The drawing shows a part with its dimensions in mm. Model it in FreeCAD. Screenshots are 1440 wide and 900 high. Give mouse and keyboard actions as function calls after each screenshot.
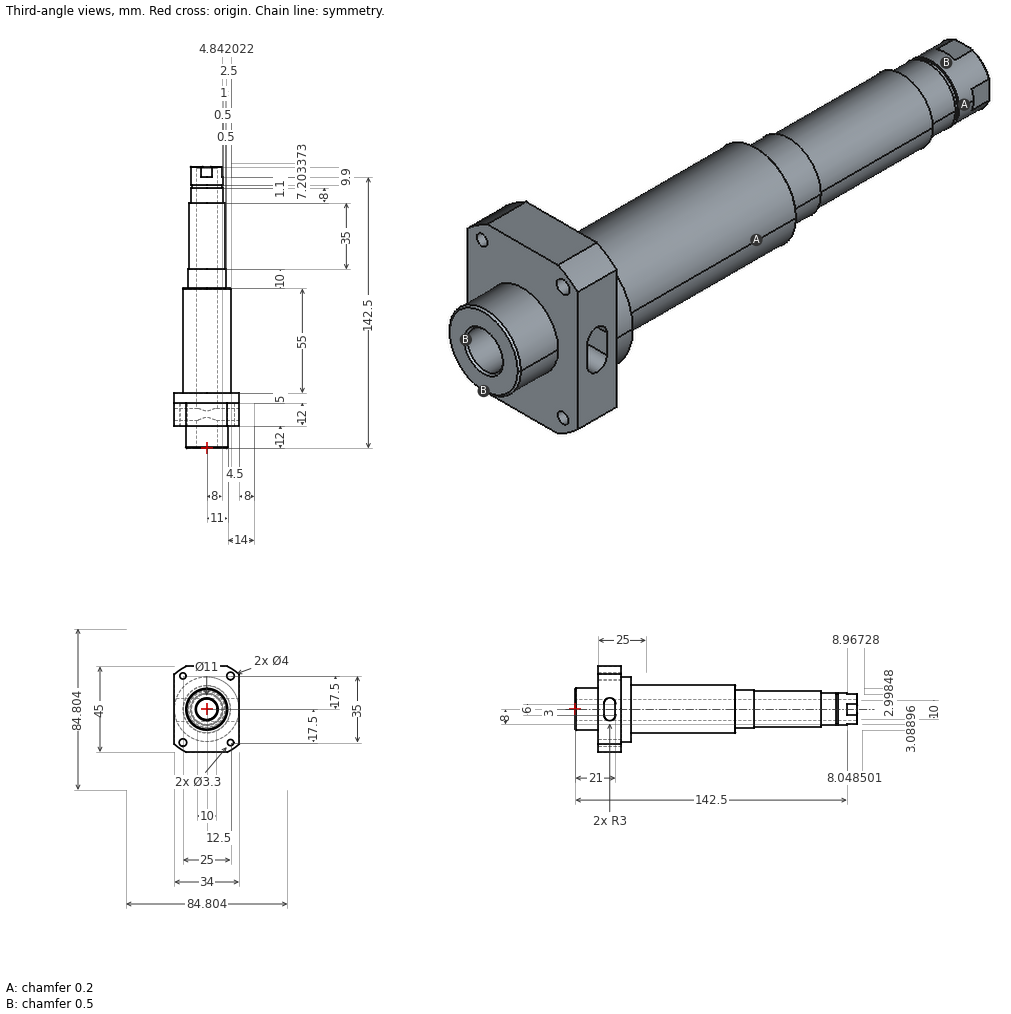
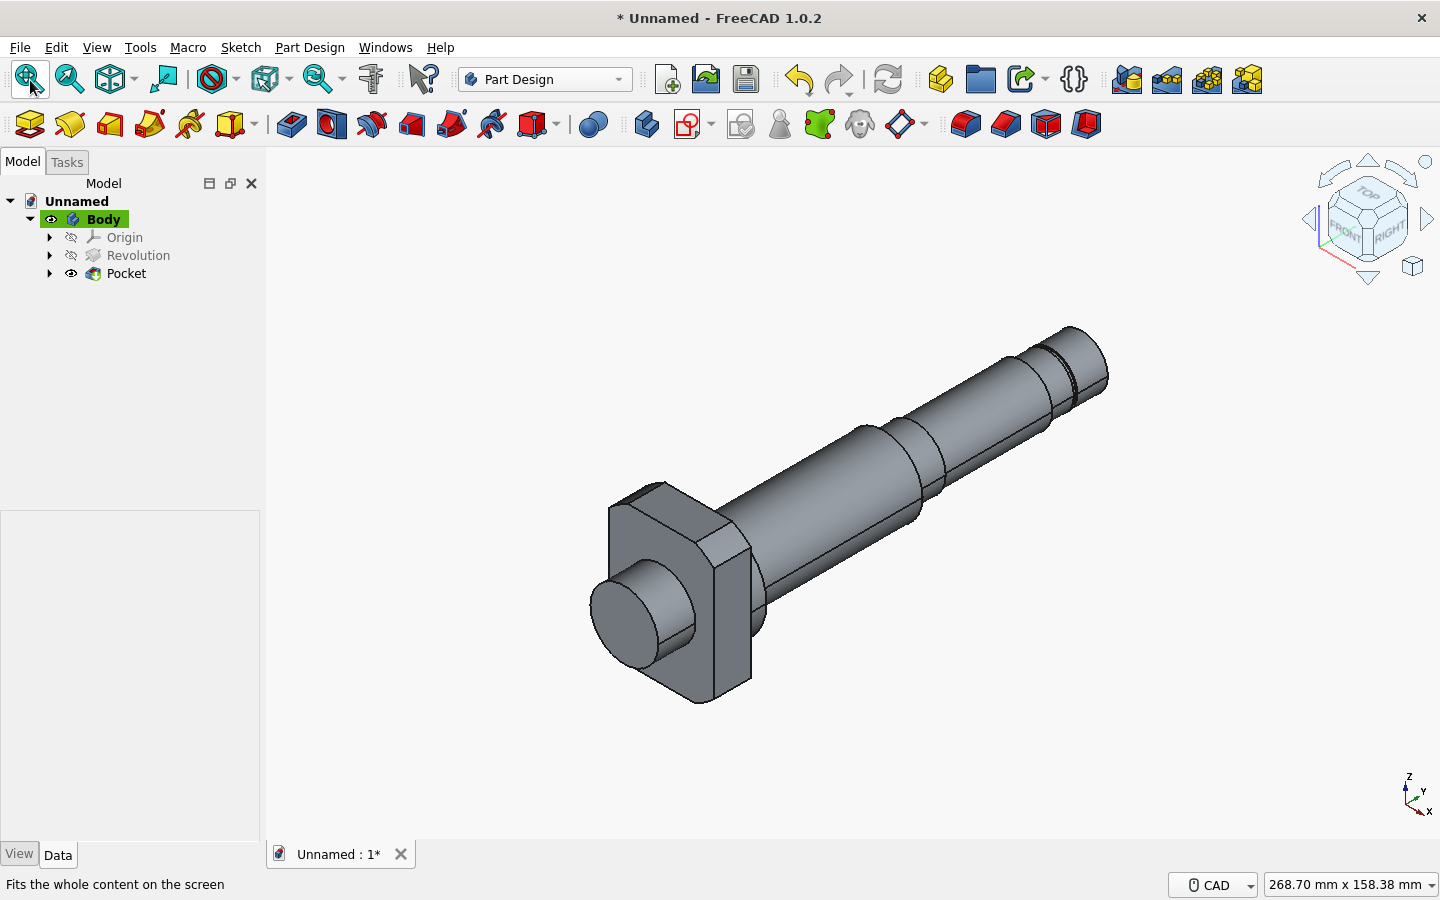
click(631, 539)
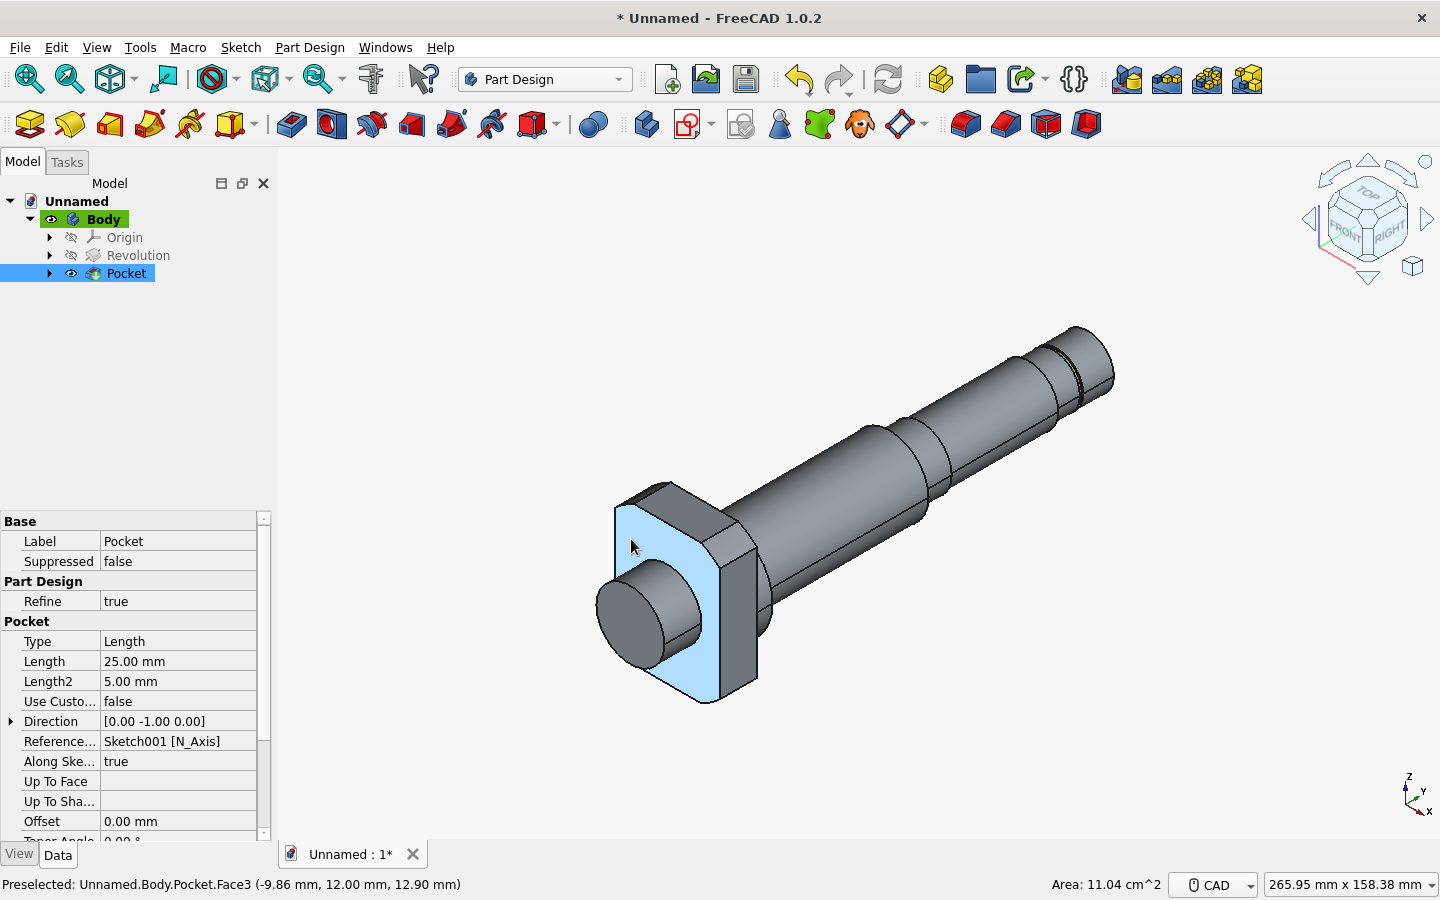
click(688, 124)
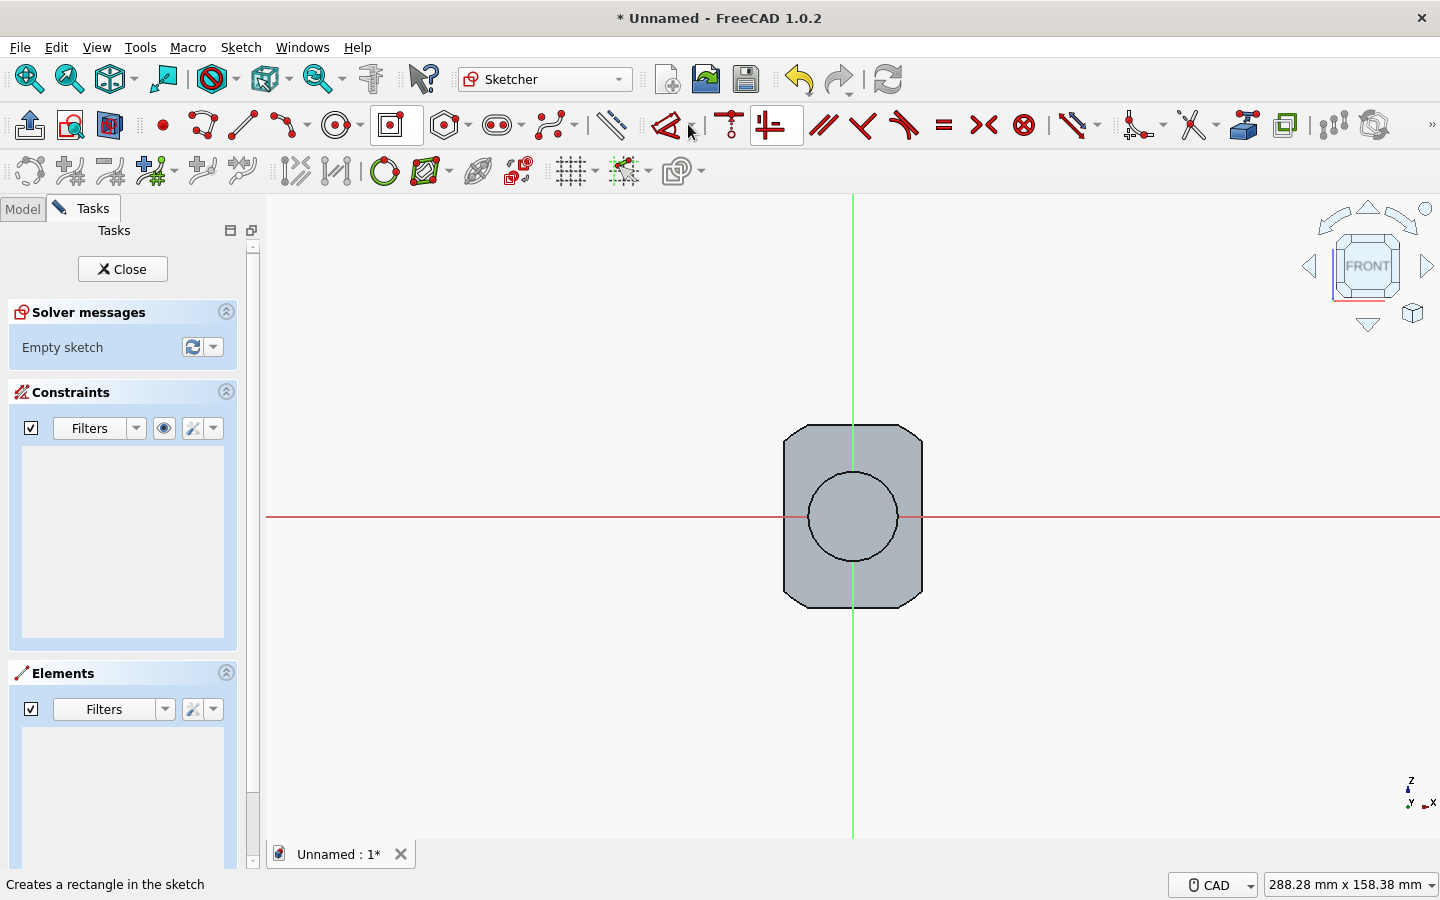
scroll(893, 516, up, 5)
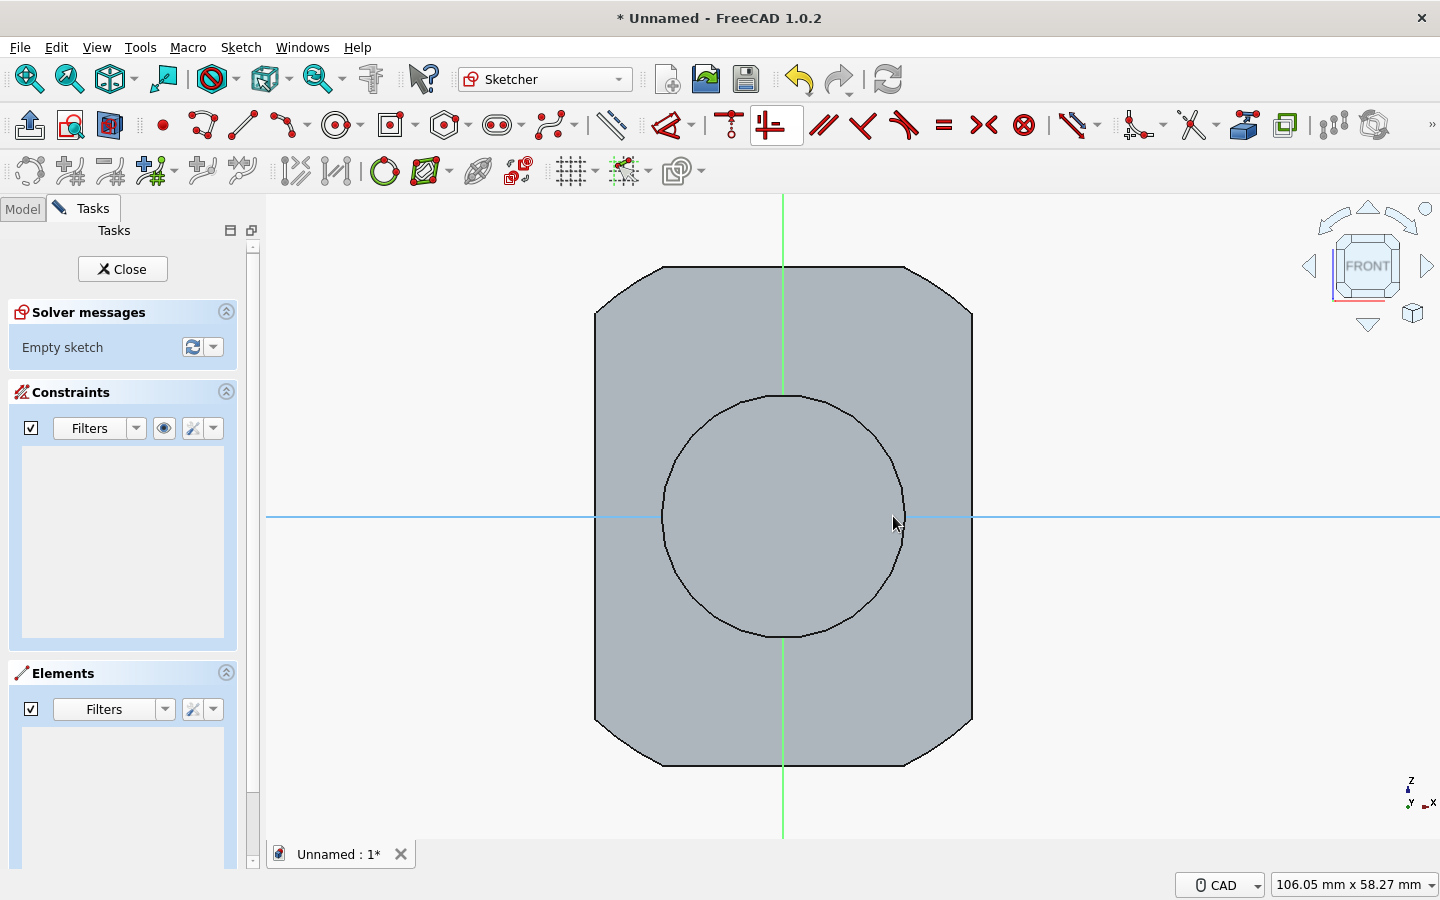
click(336, 126)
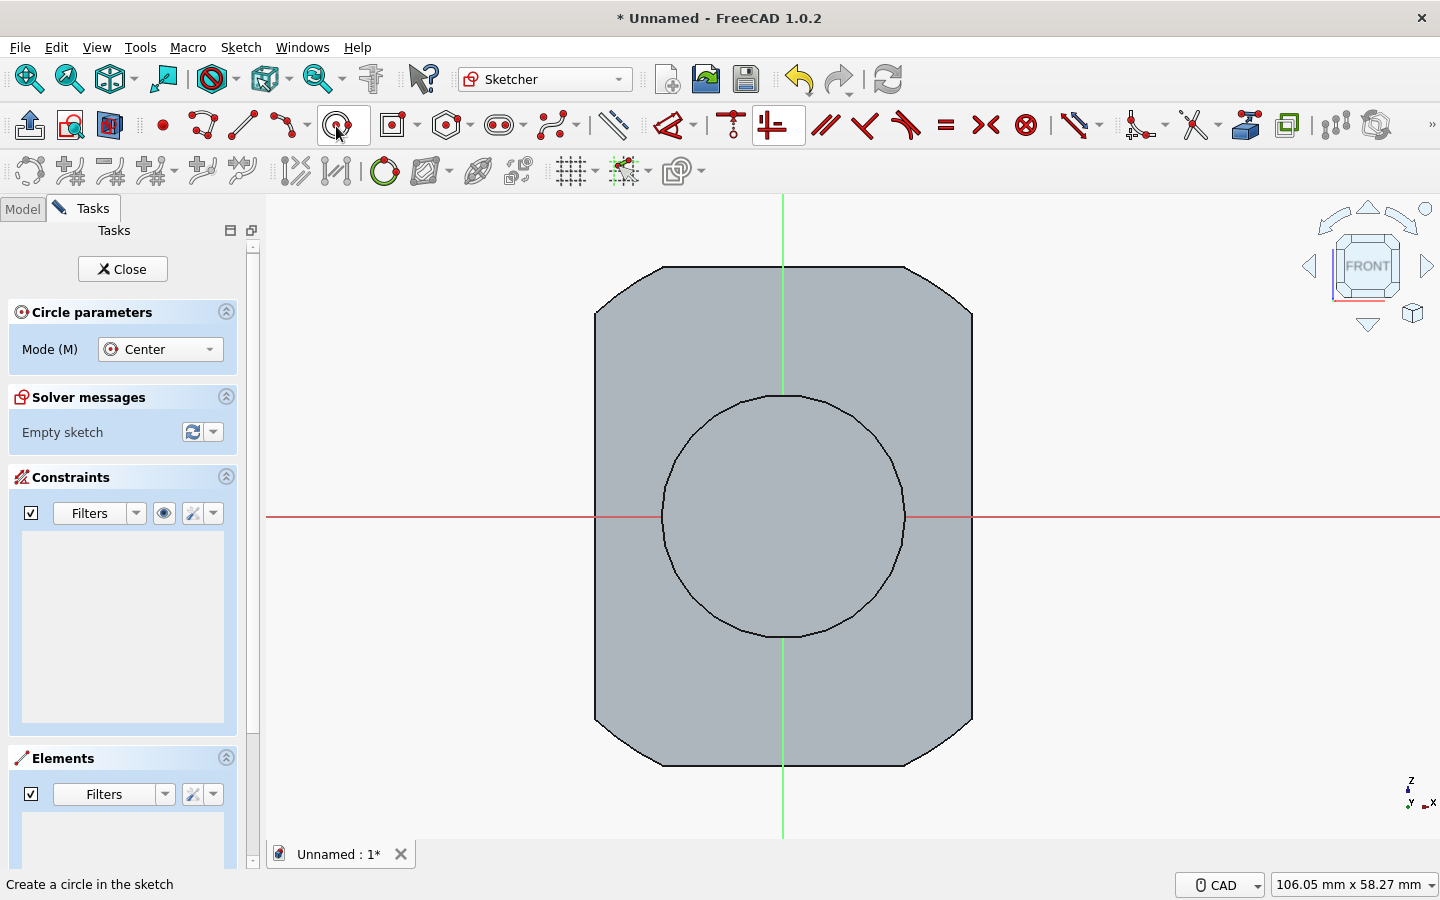
scroll(922, 710, up, 2)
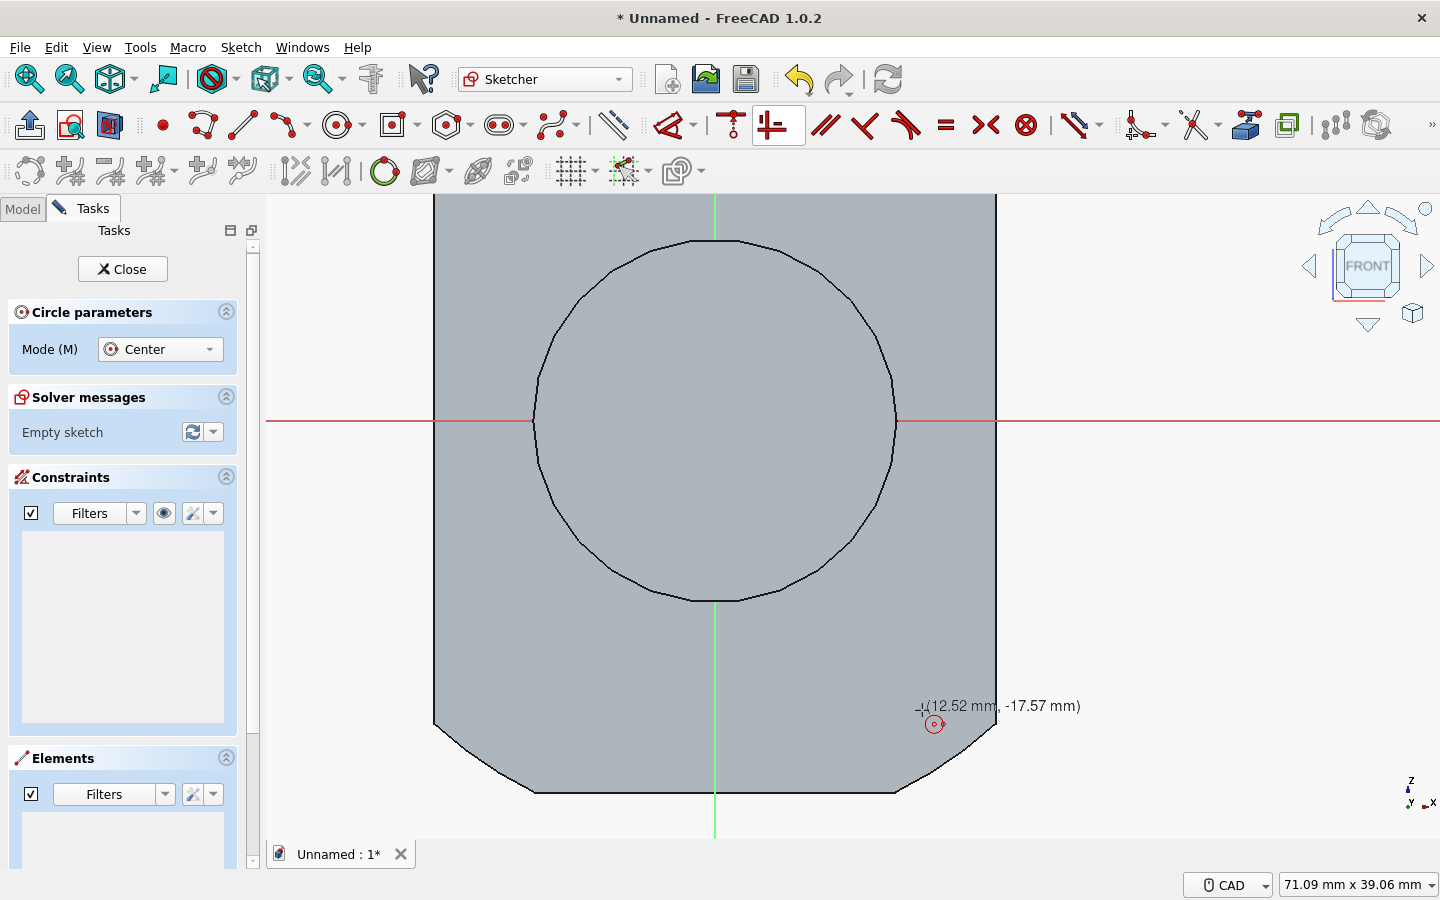
click(921, 710)
move(941, 691)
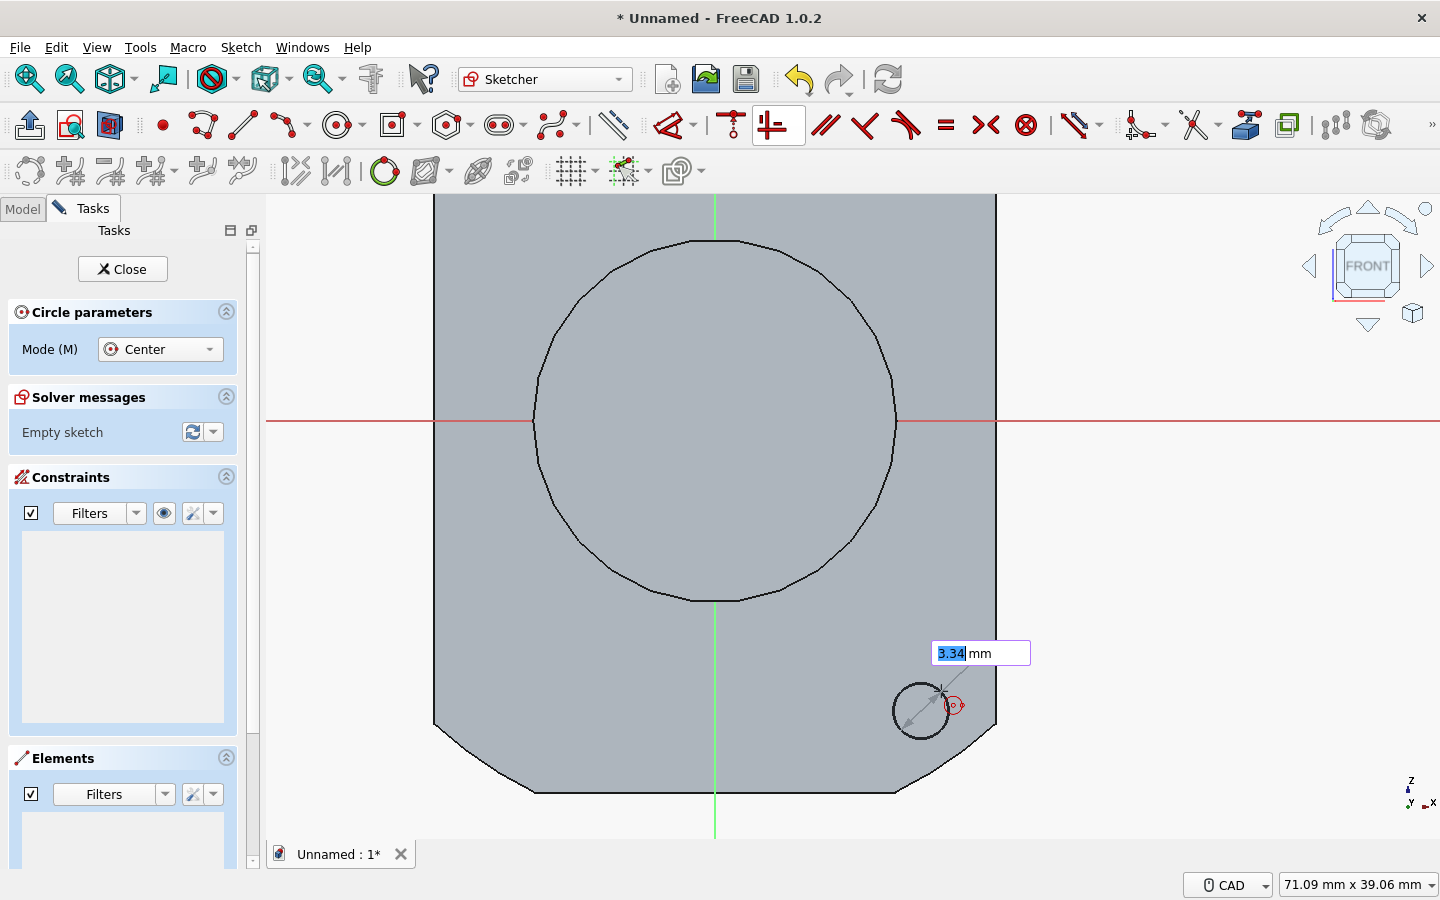
text(3.3)
key(Return)